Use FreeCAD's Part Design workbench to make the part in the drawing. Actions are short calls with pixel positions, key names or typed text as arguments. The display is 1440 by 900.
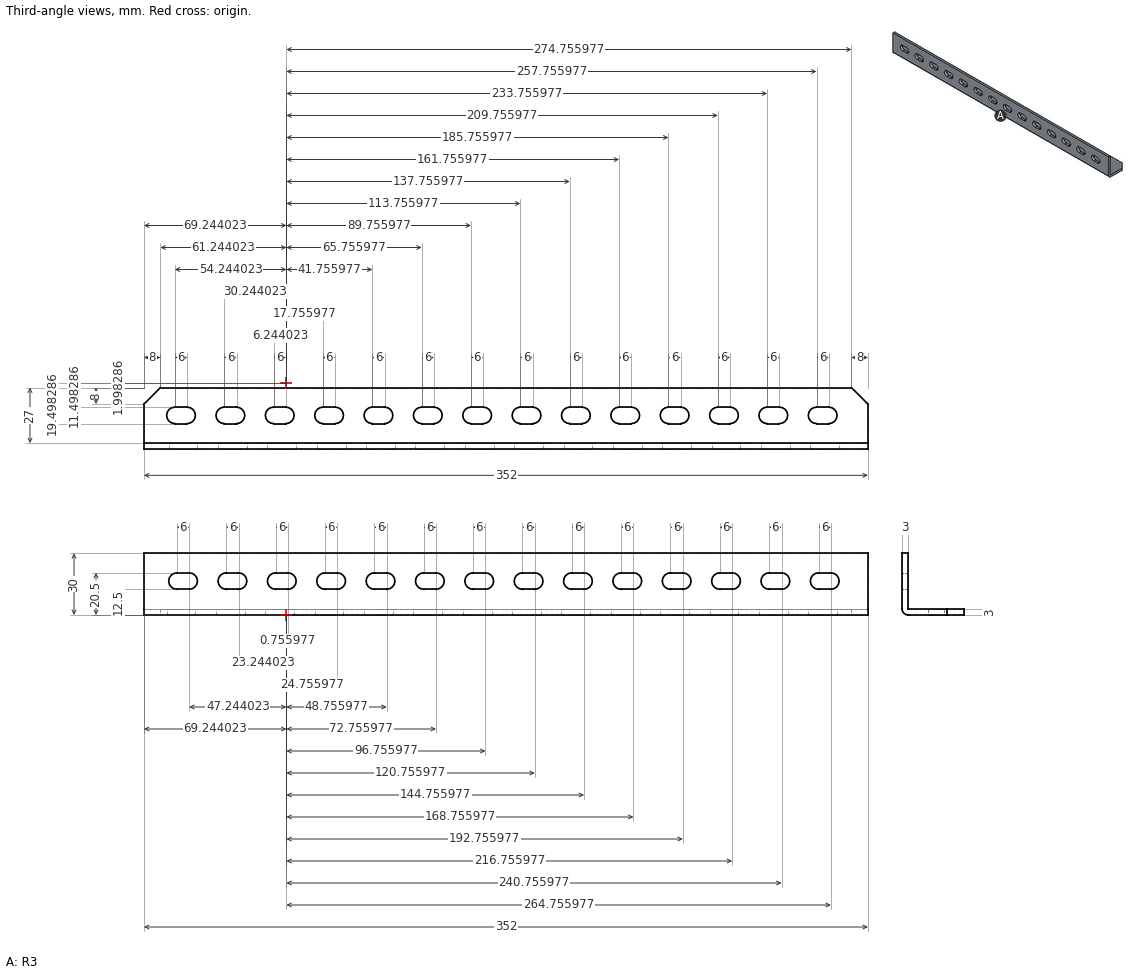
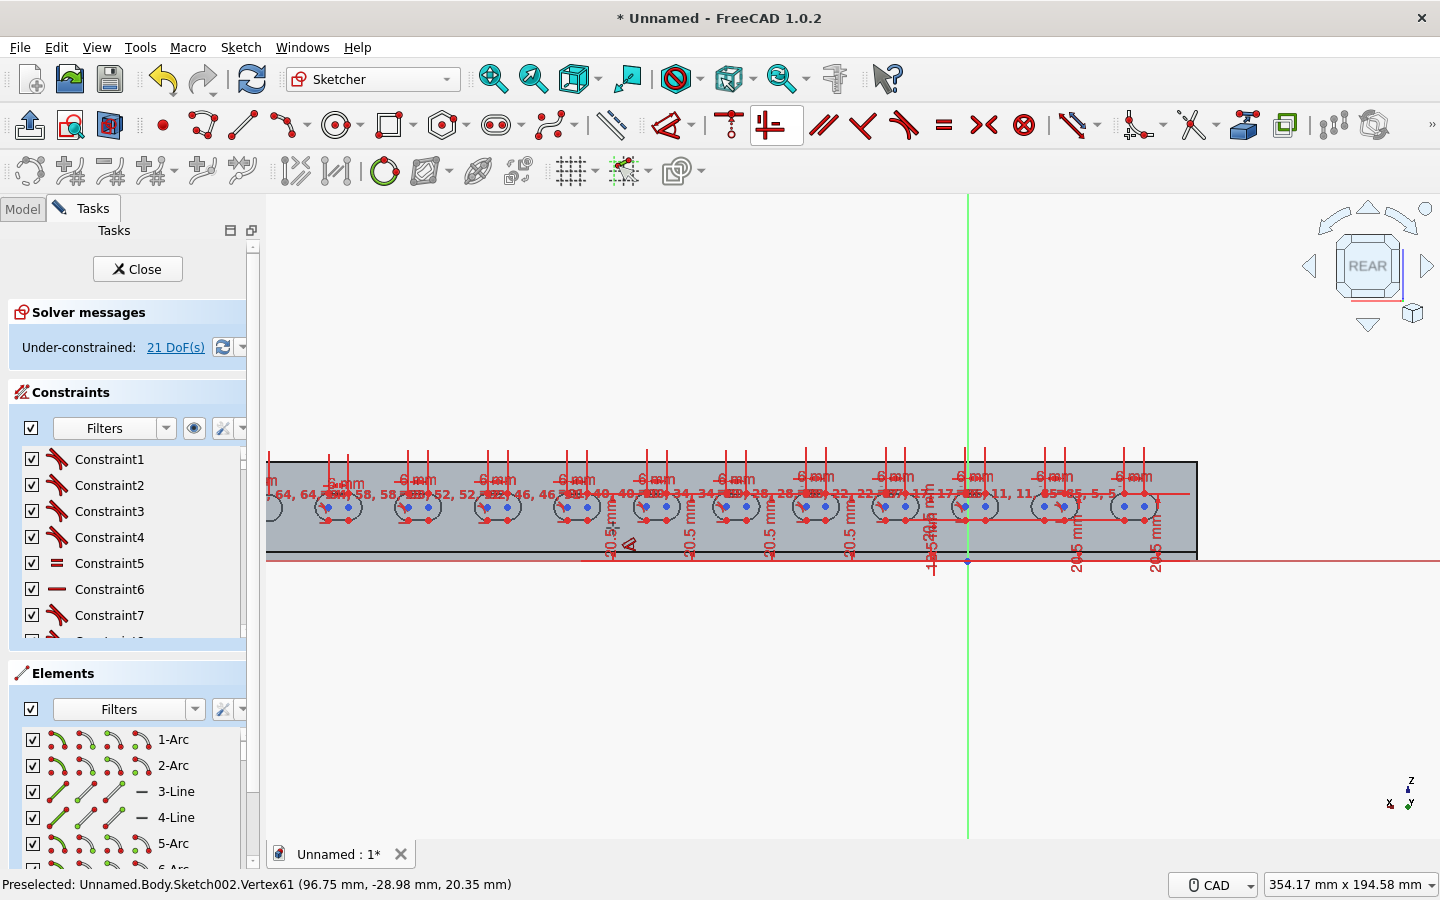
click(567, 494)
click(533, 528)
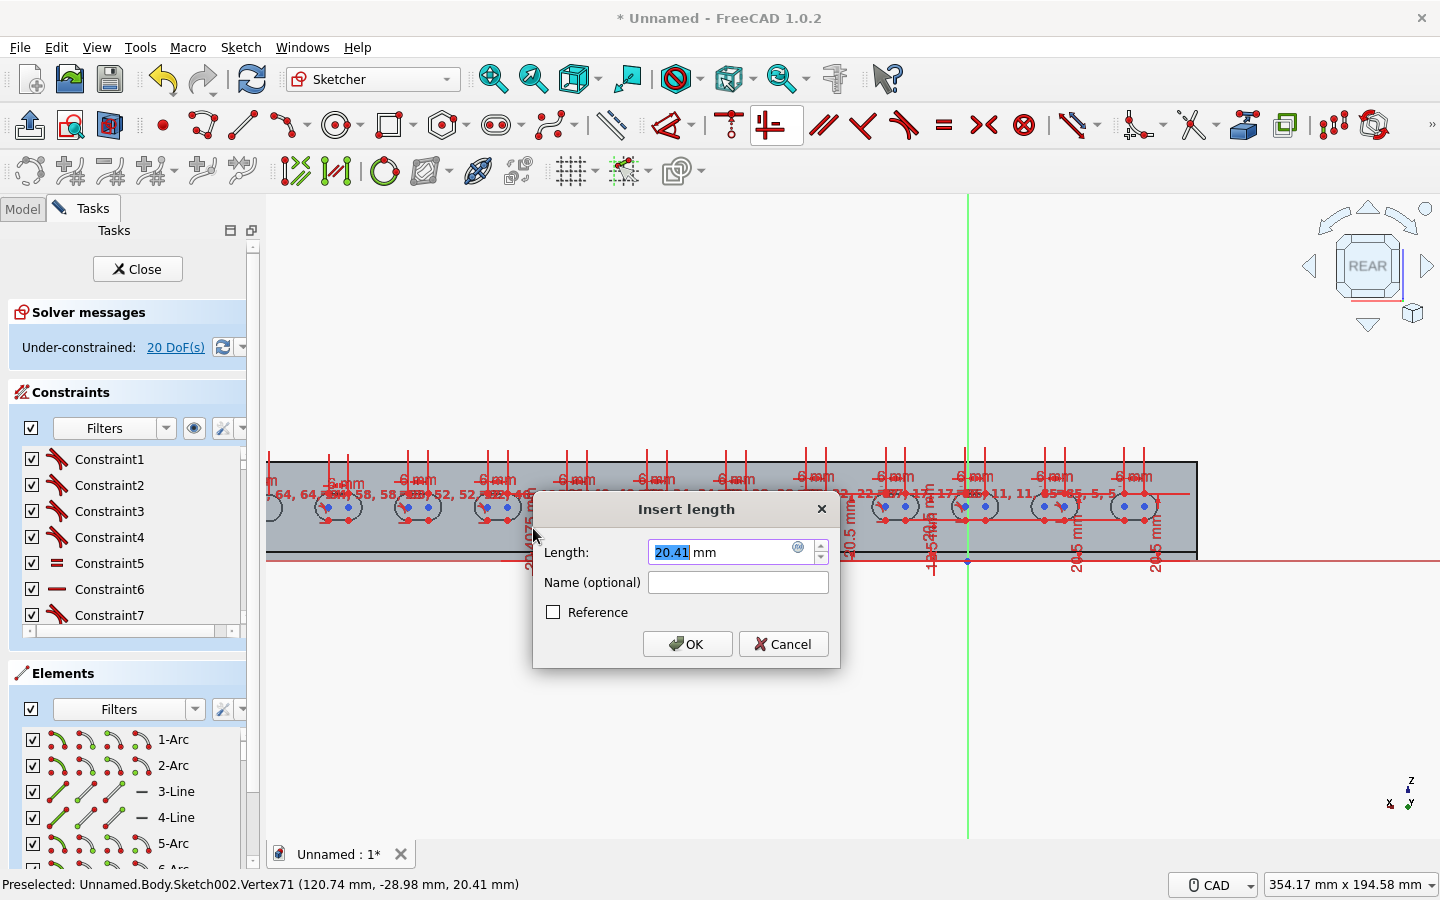
text(20.5)
key(Return)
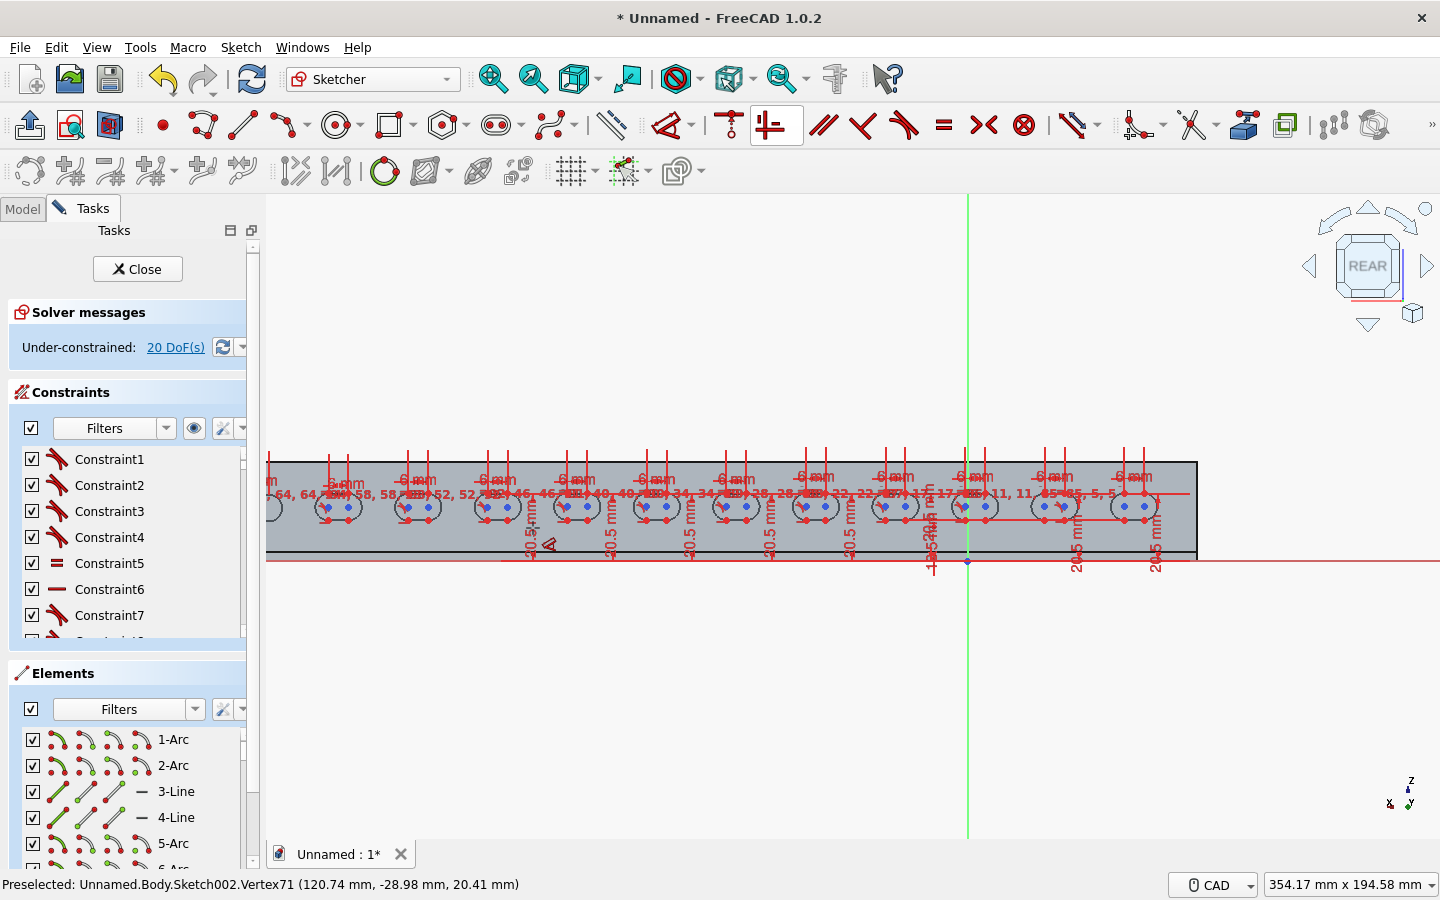
click(488, 494)
click(454, 528)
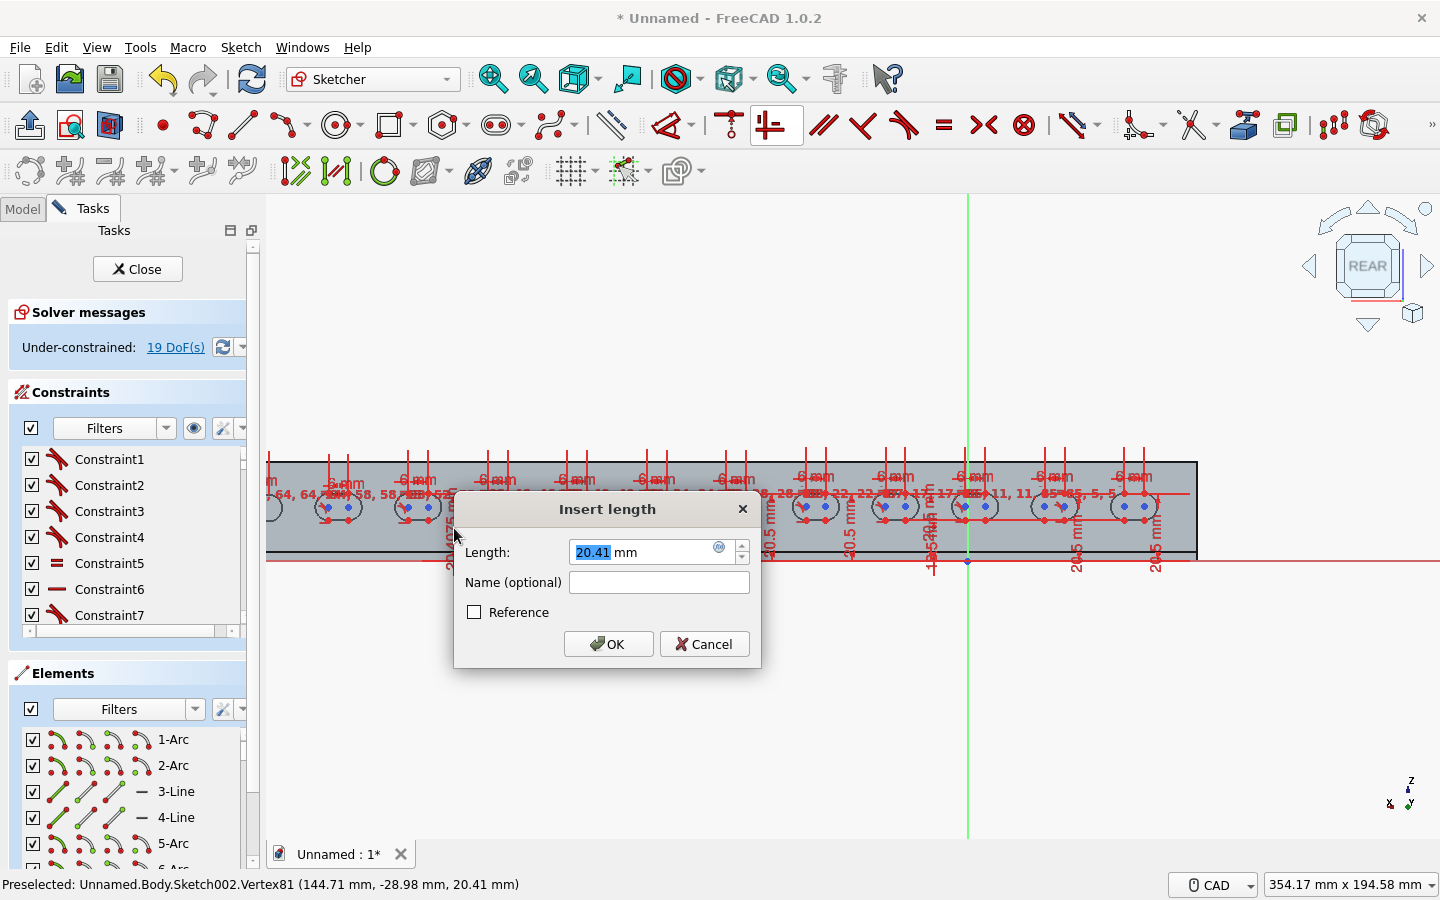
text(20.5)
key(Return)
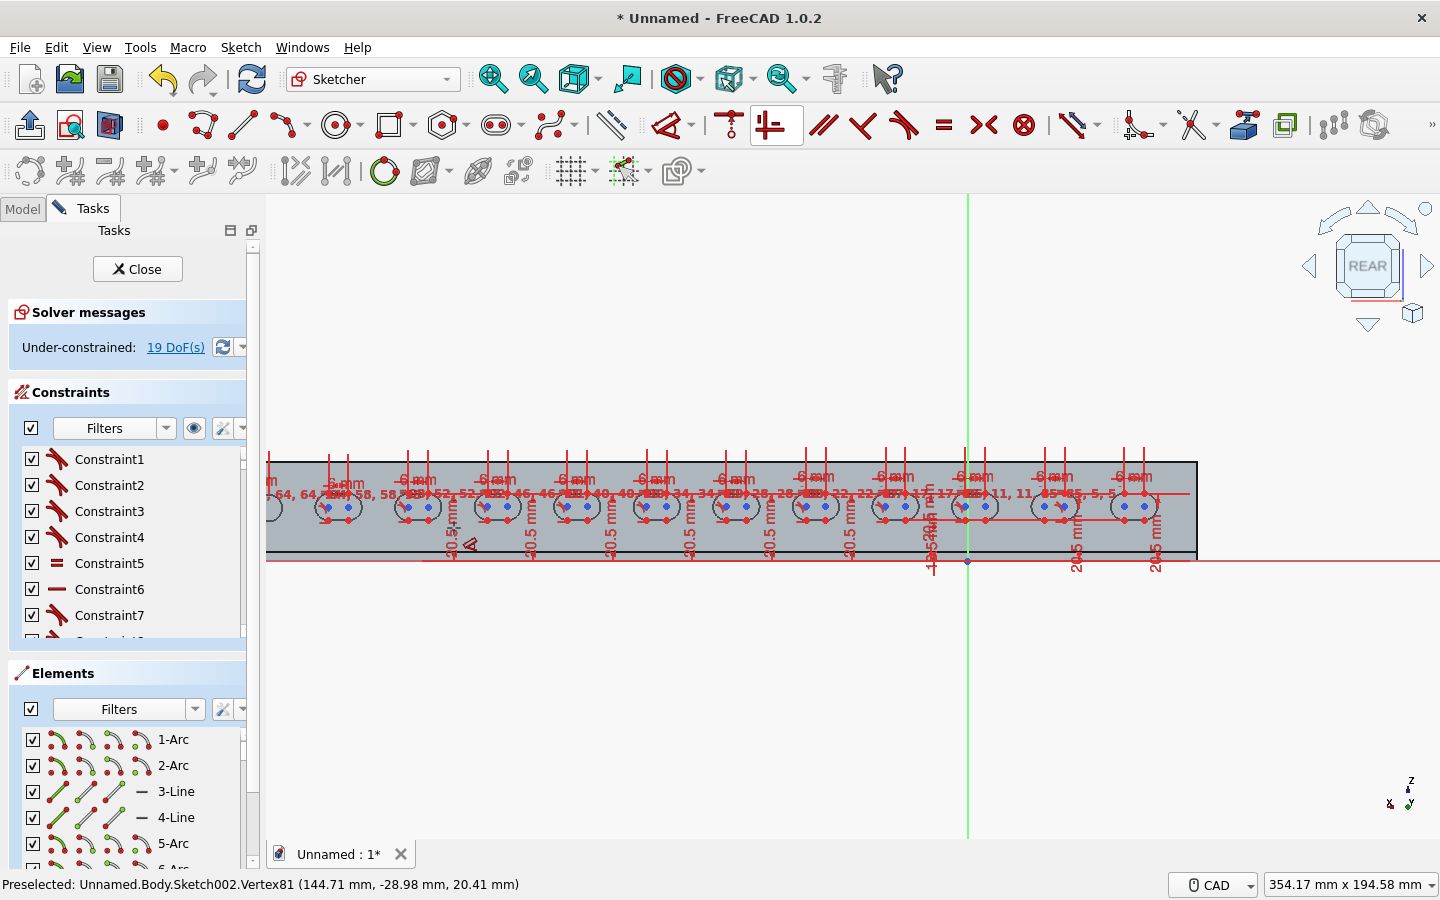
click(408, 494)
click(374, 528)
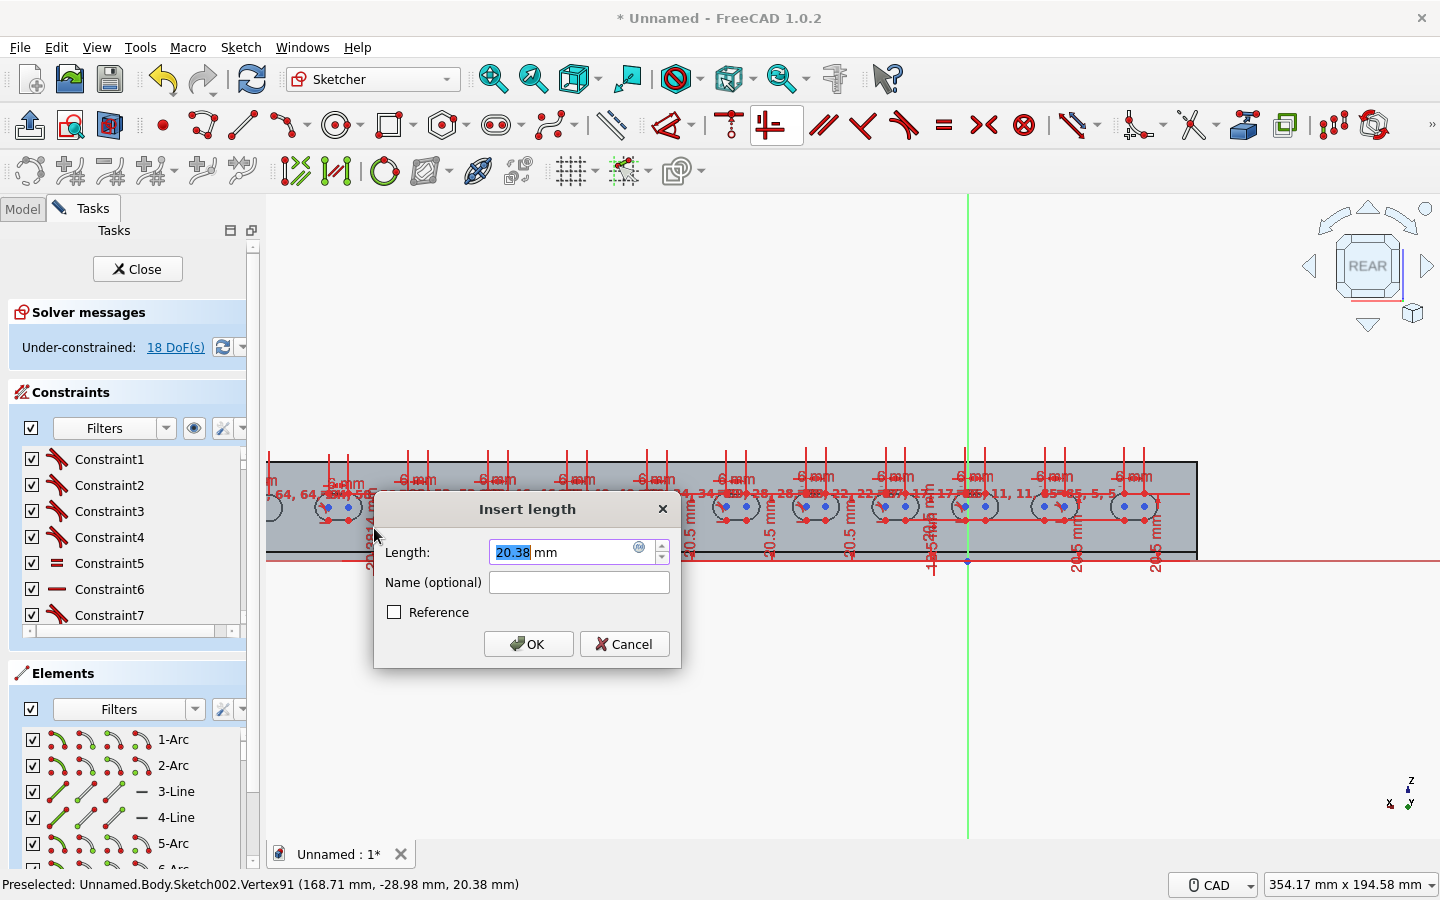
text(20.5)
key(Return)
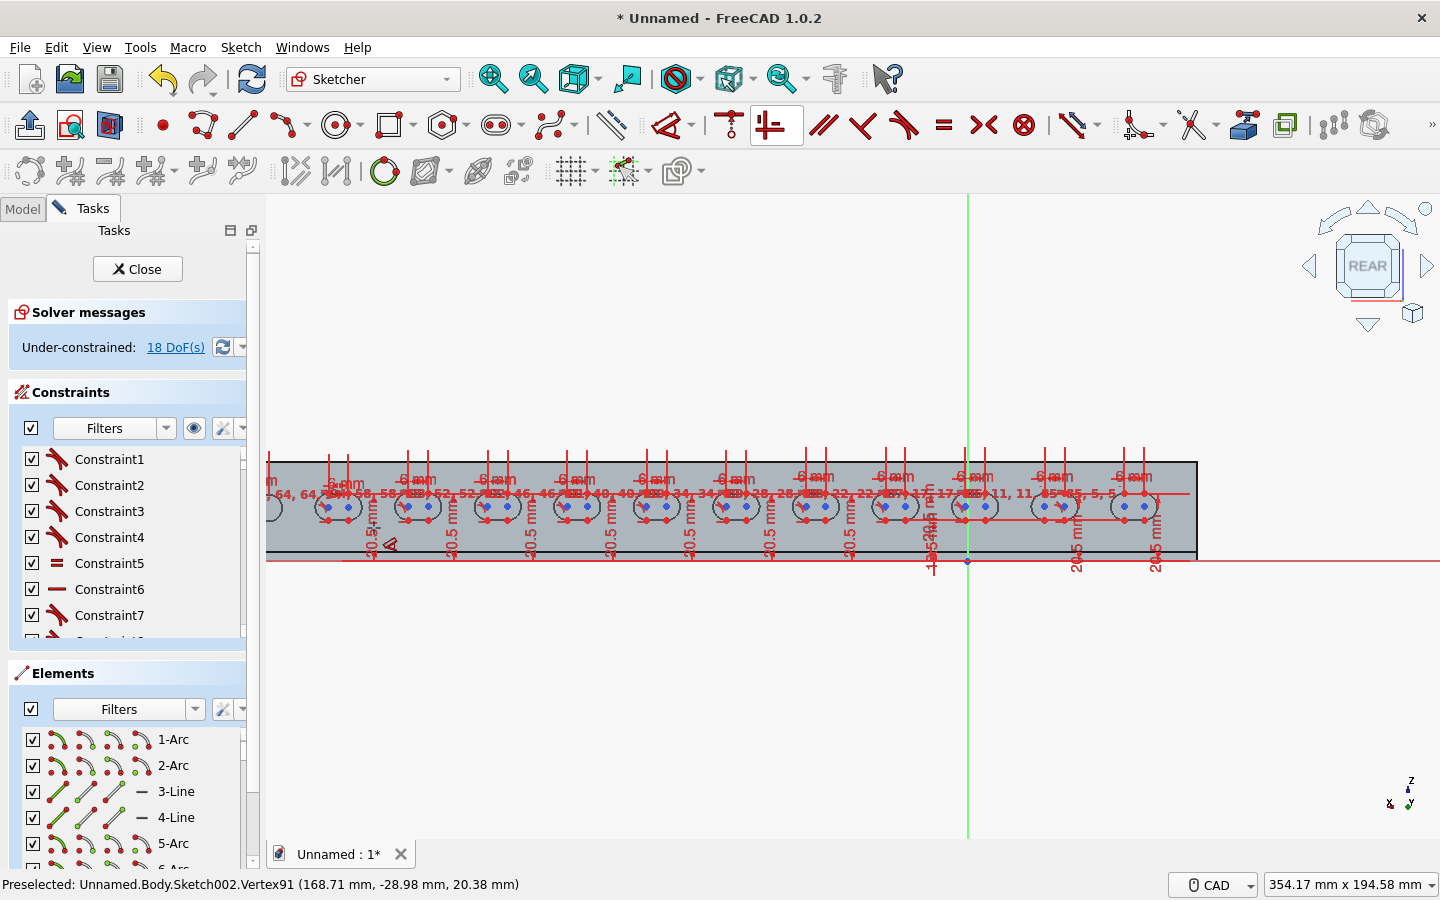
click(329, 494)
click(295, 528)